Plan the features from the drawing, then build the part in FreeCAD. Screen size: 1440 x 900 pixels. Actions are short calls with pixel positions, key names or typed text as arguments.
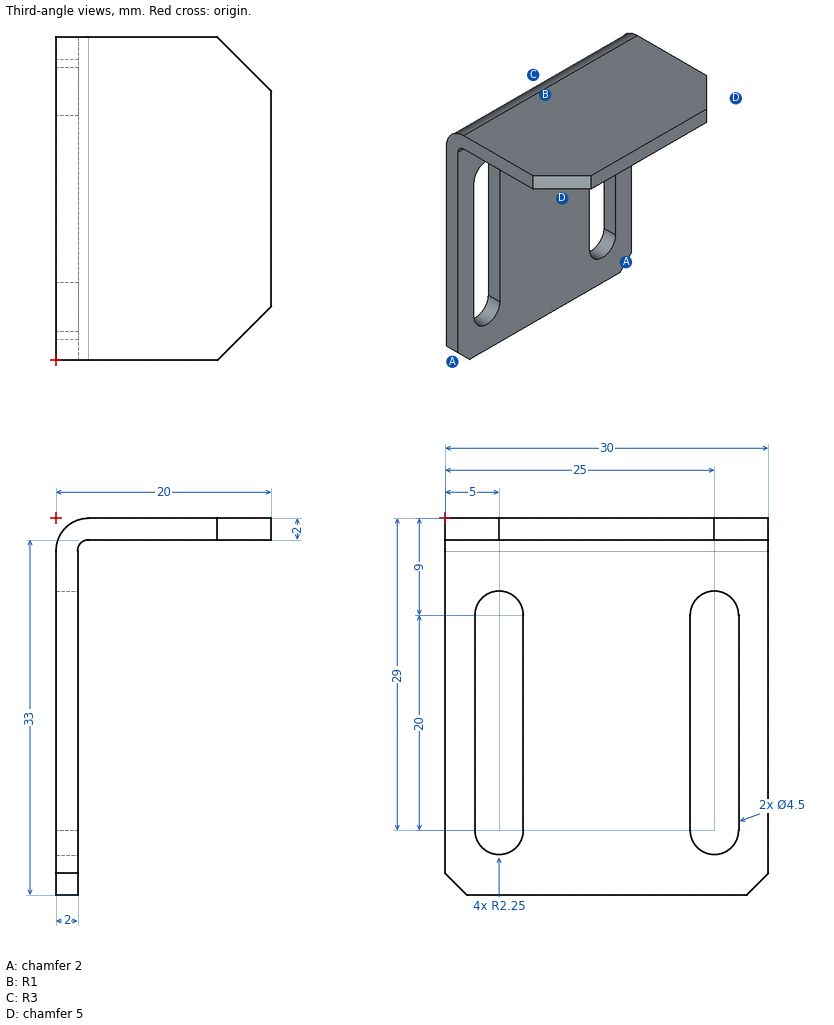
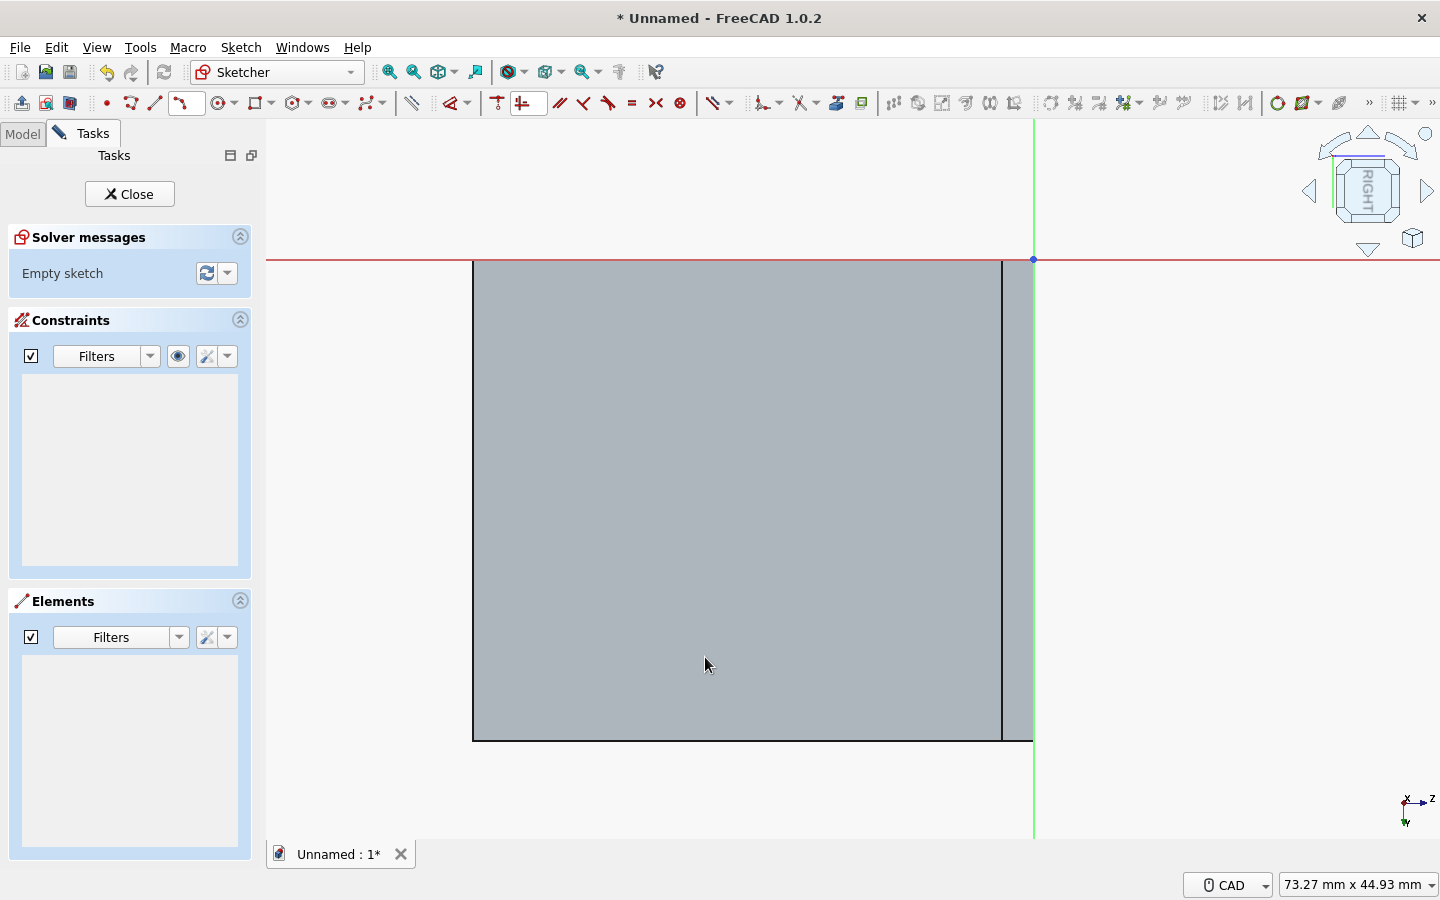
click(218, 104)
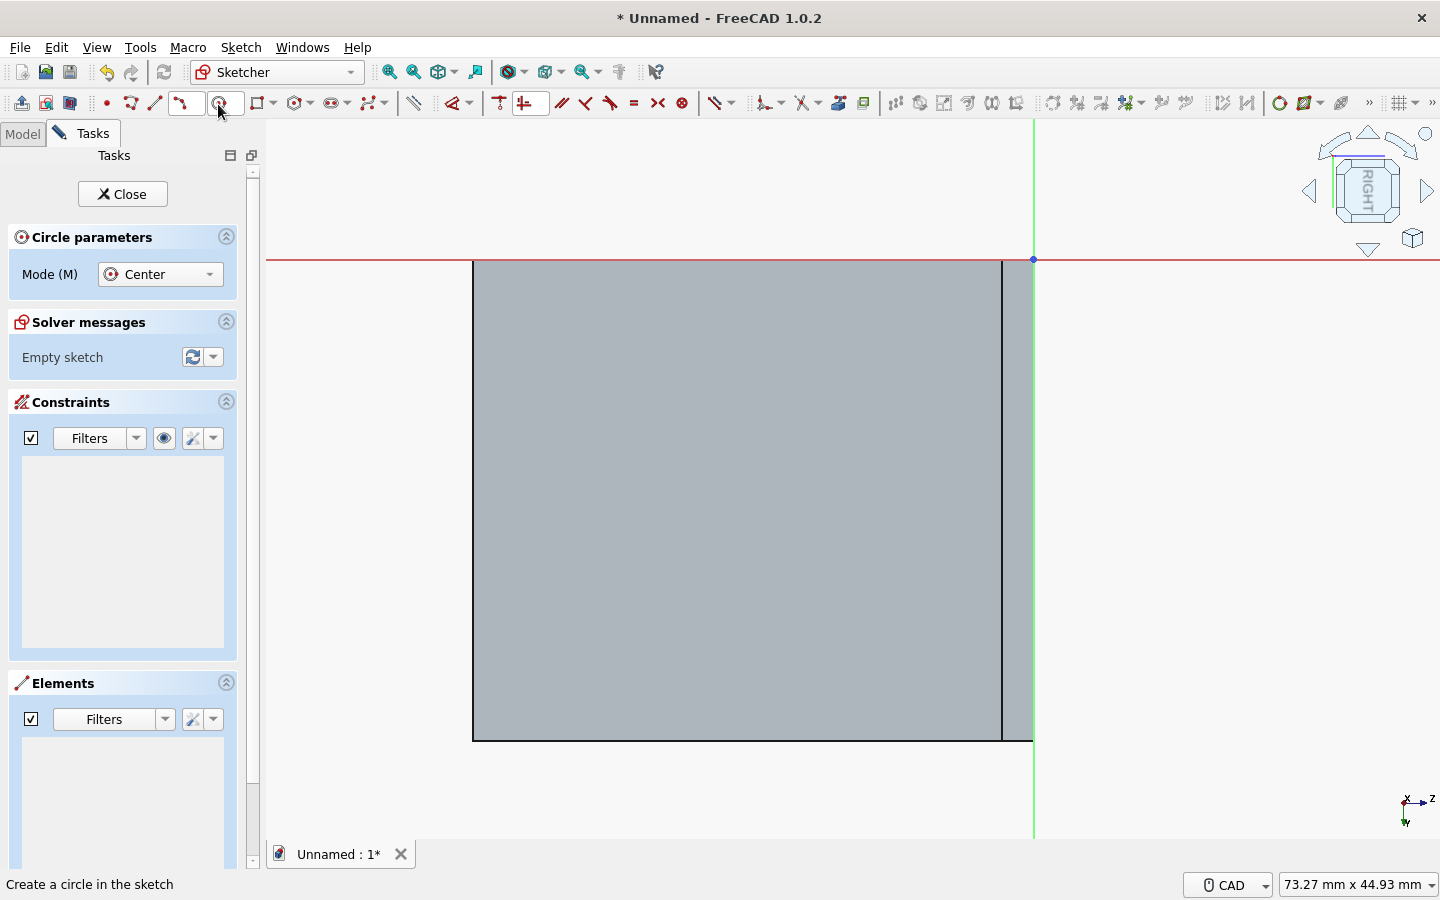
click(569, 661)
move(595, 635)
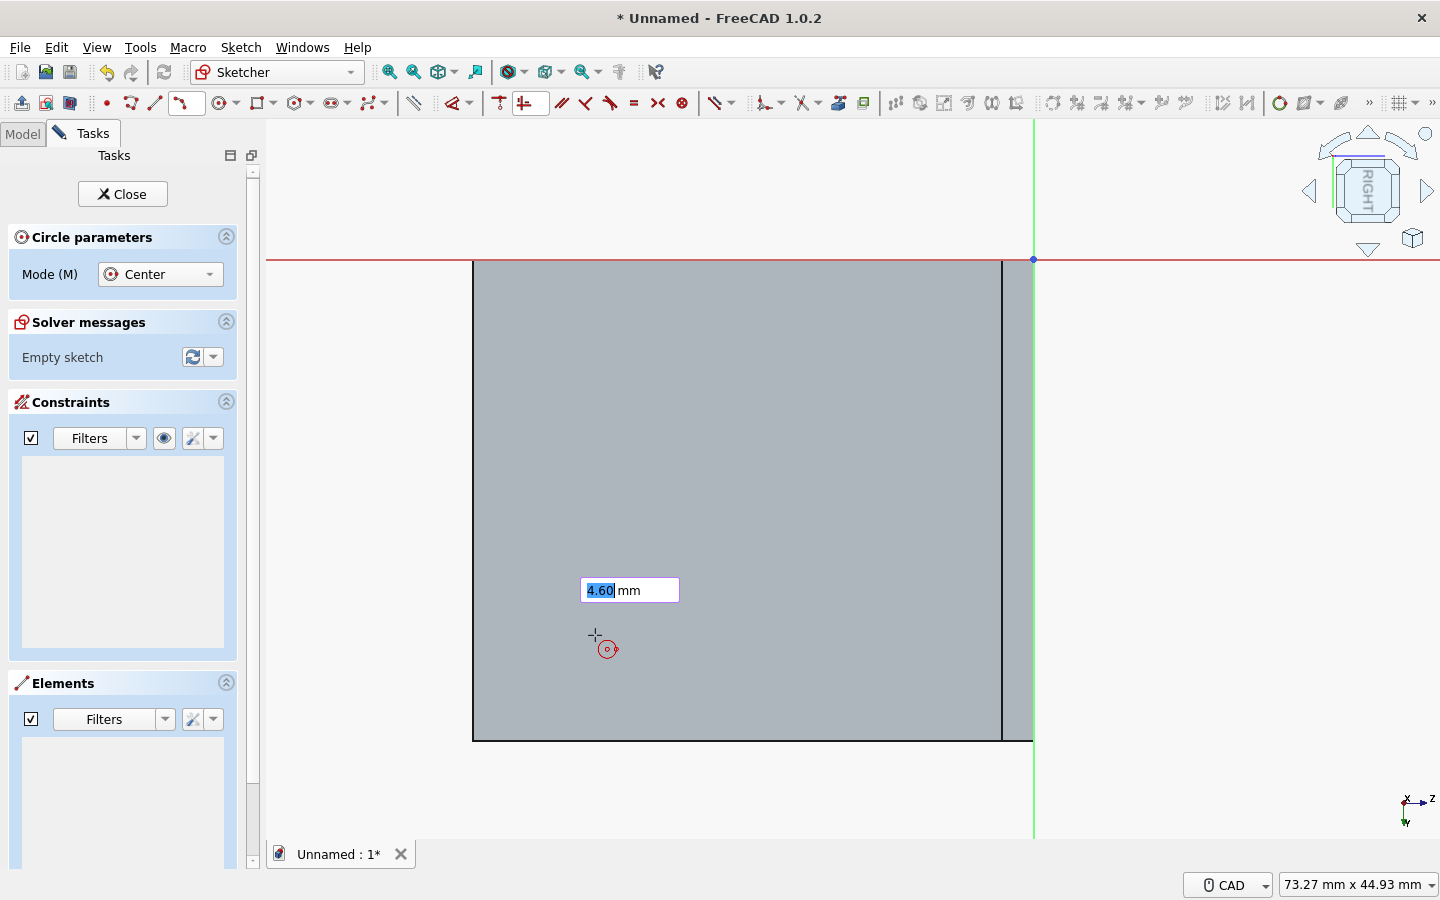
text(4.5)
key(Return)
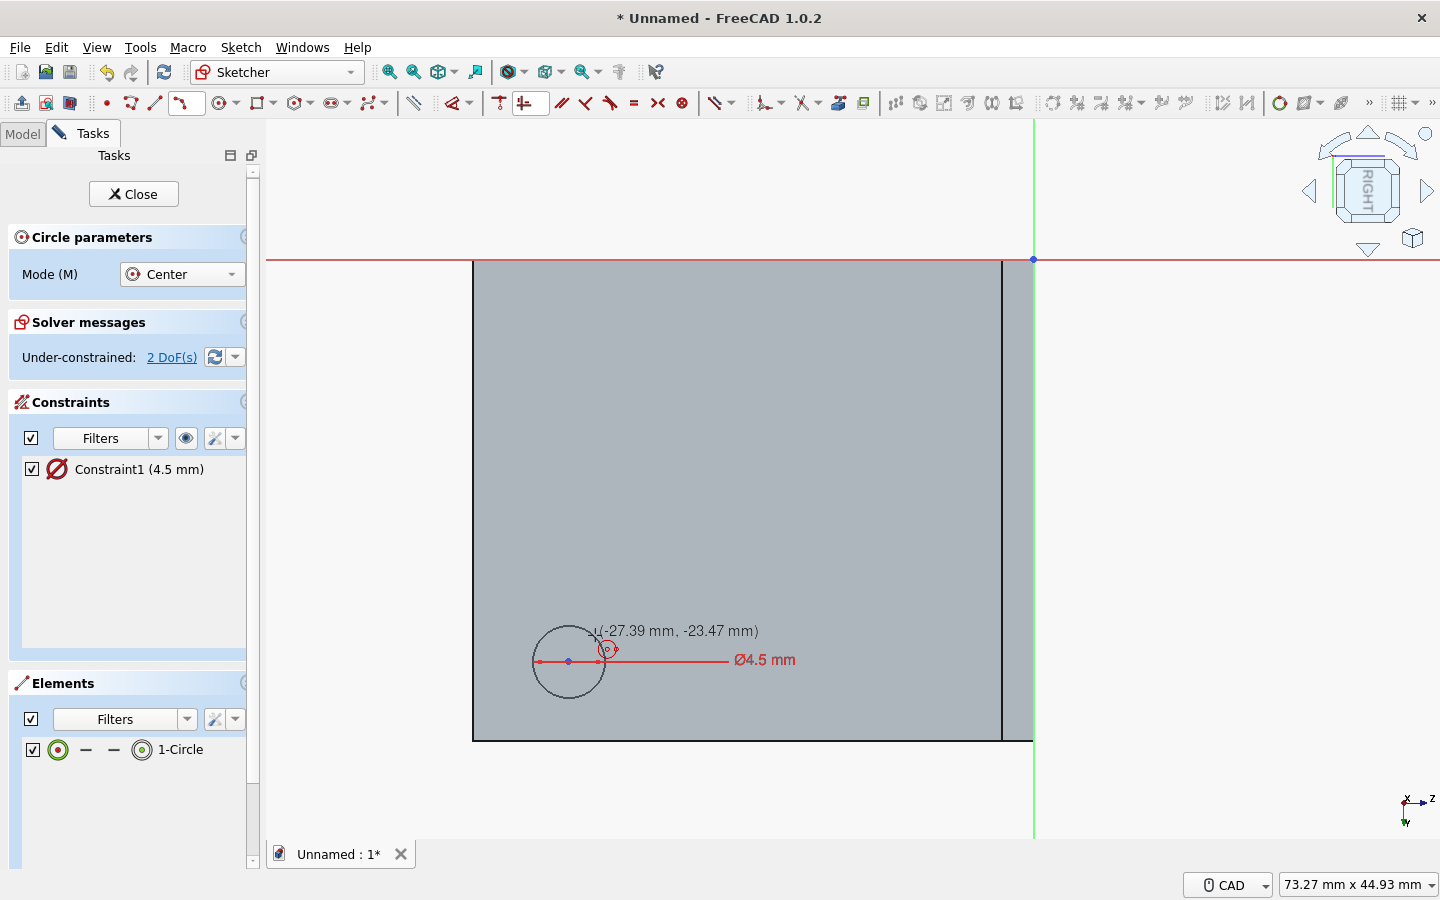
click(569, 340)
move(595, 315)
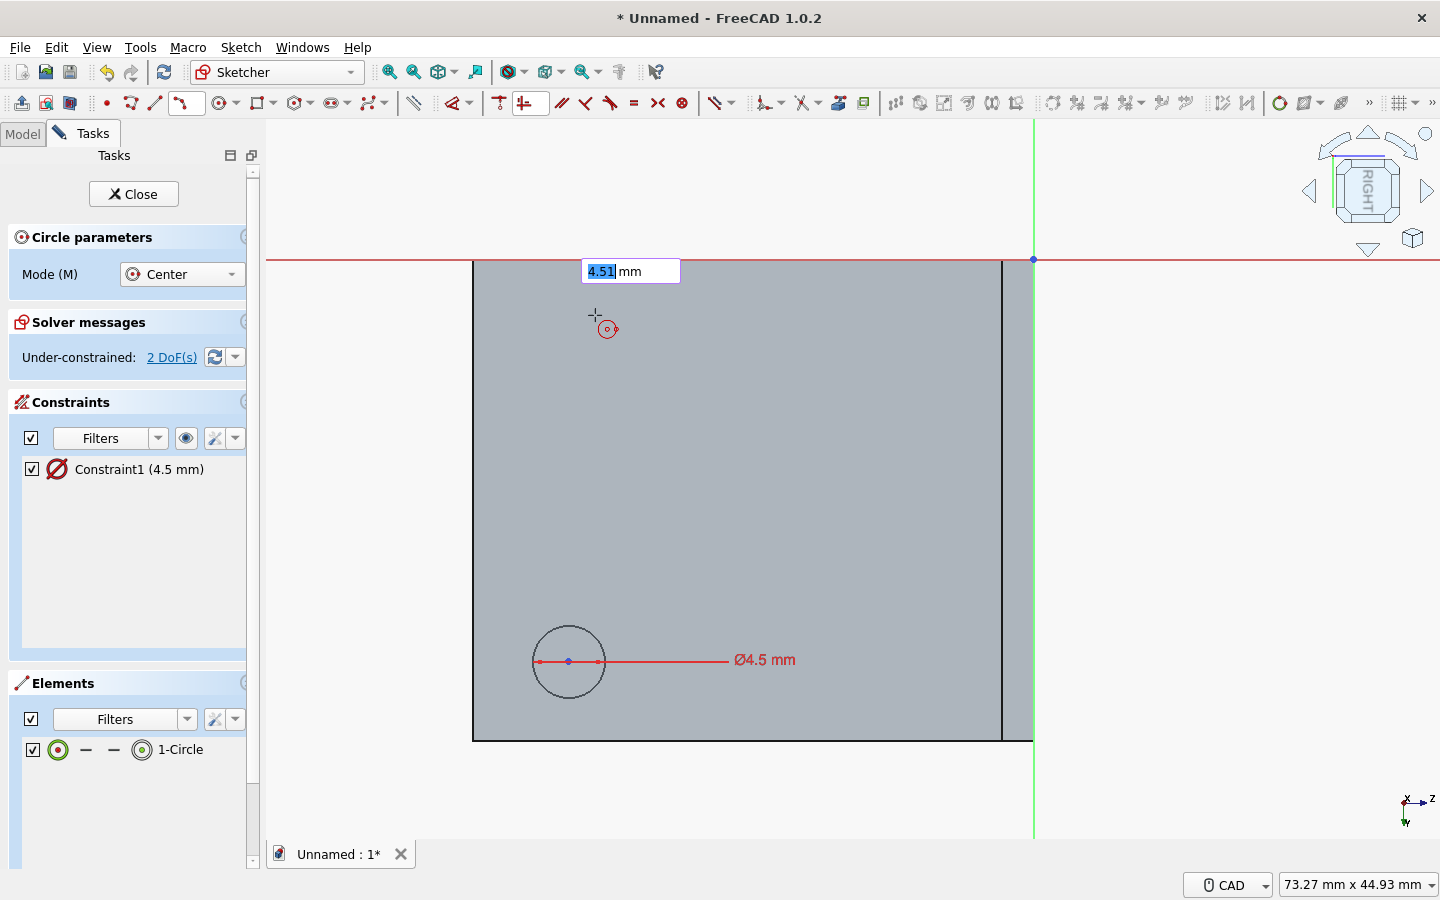
text(4.5)
key(Return)
key(Escape)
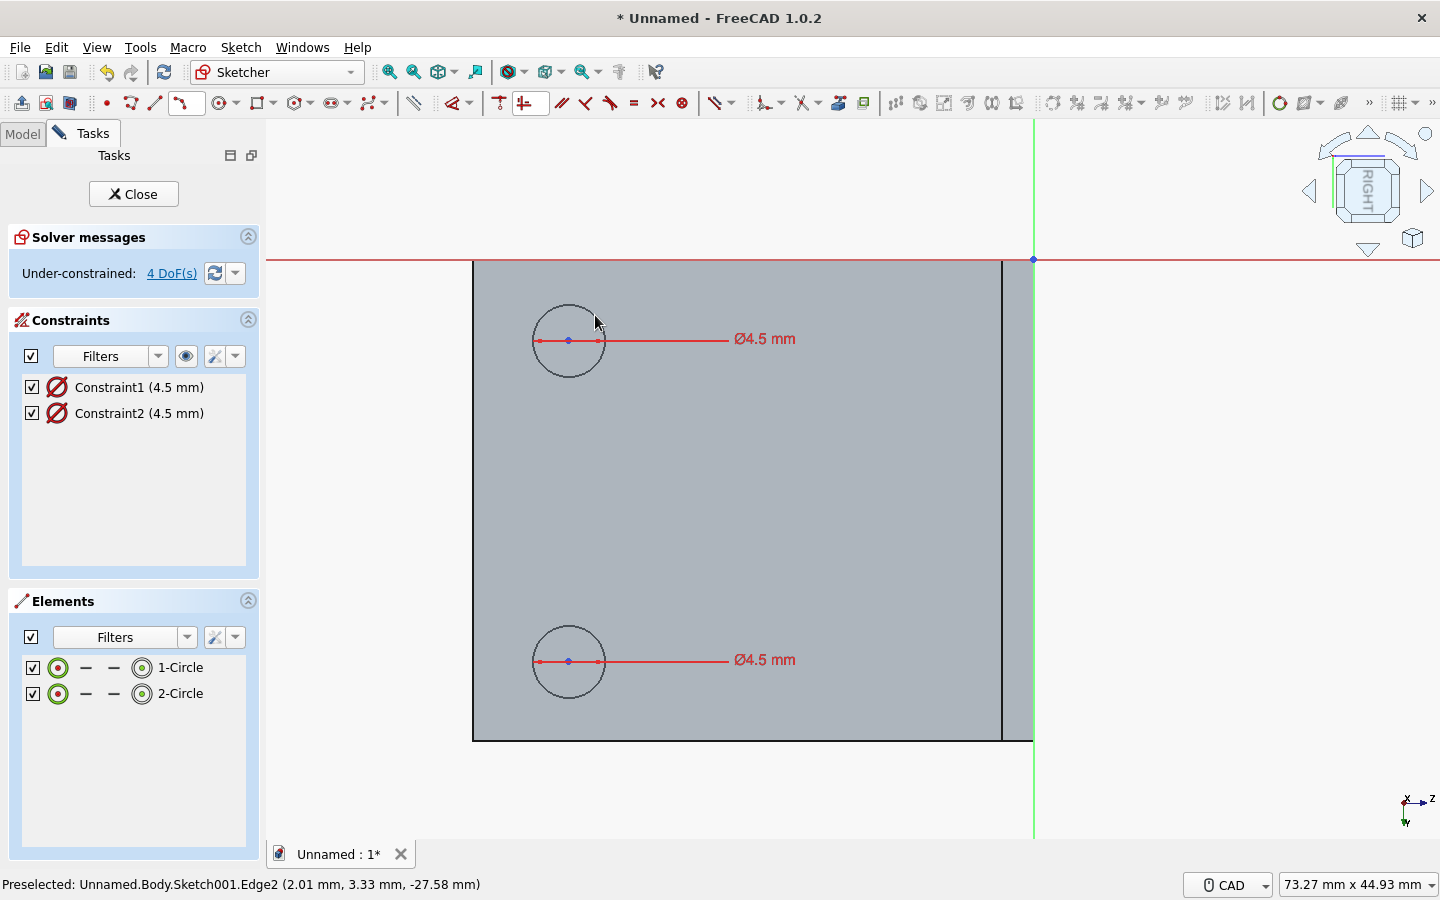
click(452, 104)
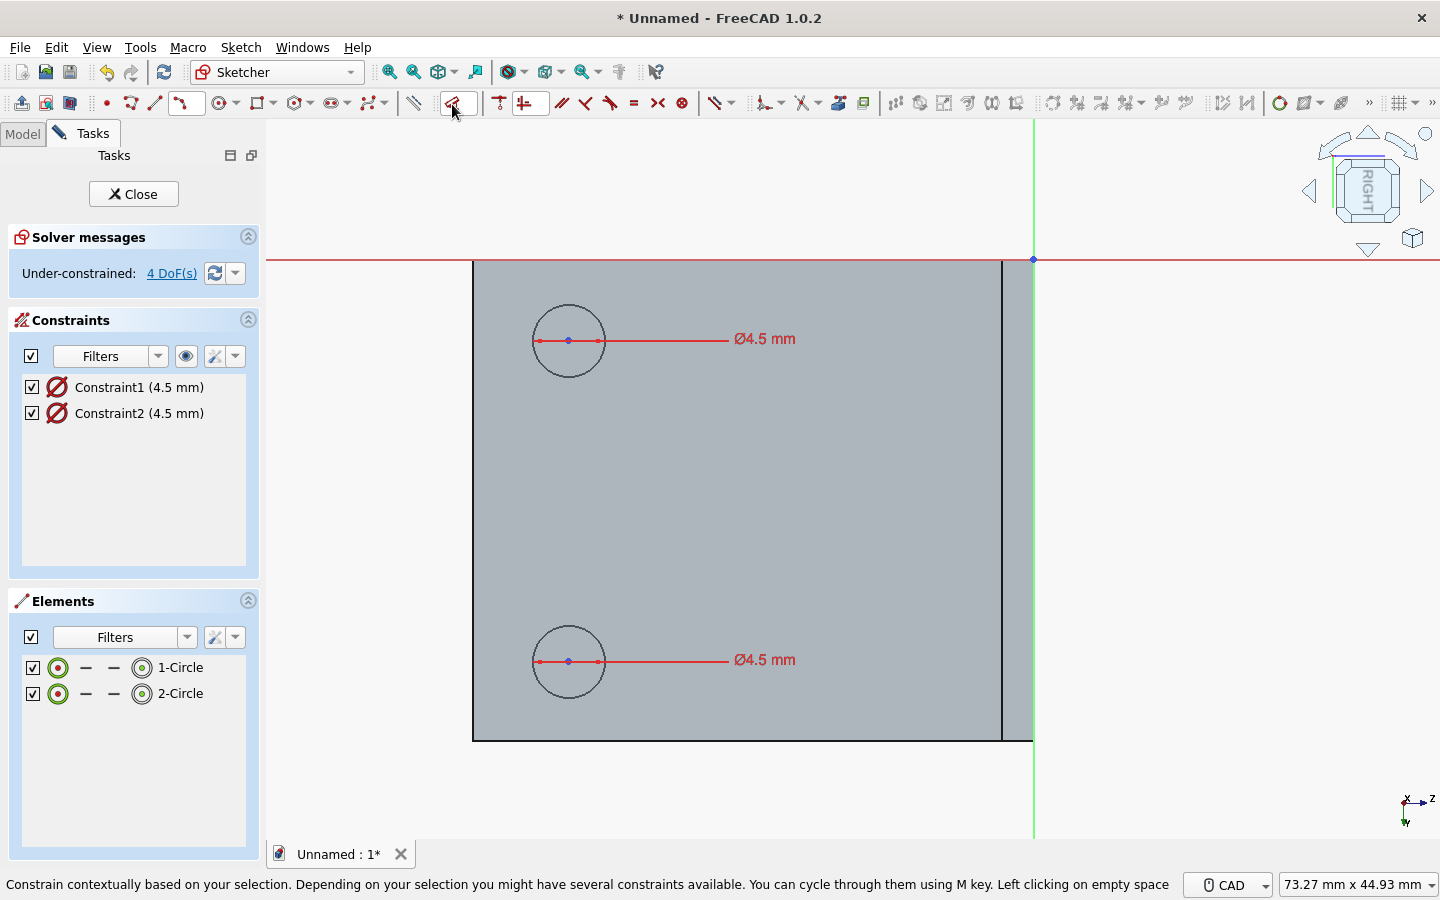
click(569, 341)
click(1068, 300)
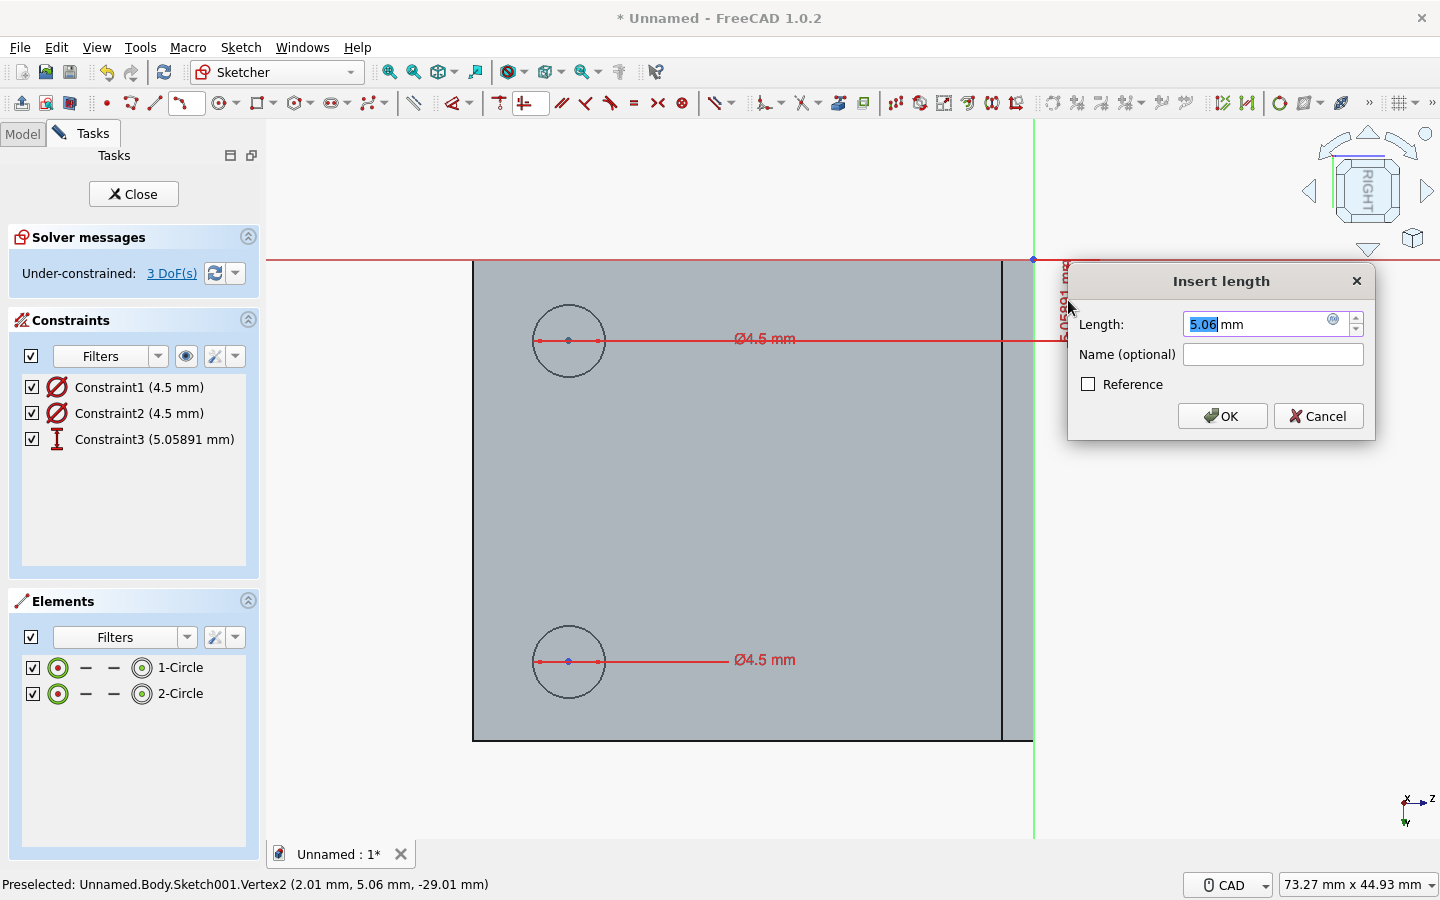
text(5)
key(Return)